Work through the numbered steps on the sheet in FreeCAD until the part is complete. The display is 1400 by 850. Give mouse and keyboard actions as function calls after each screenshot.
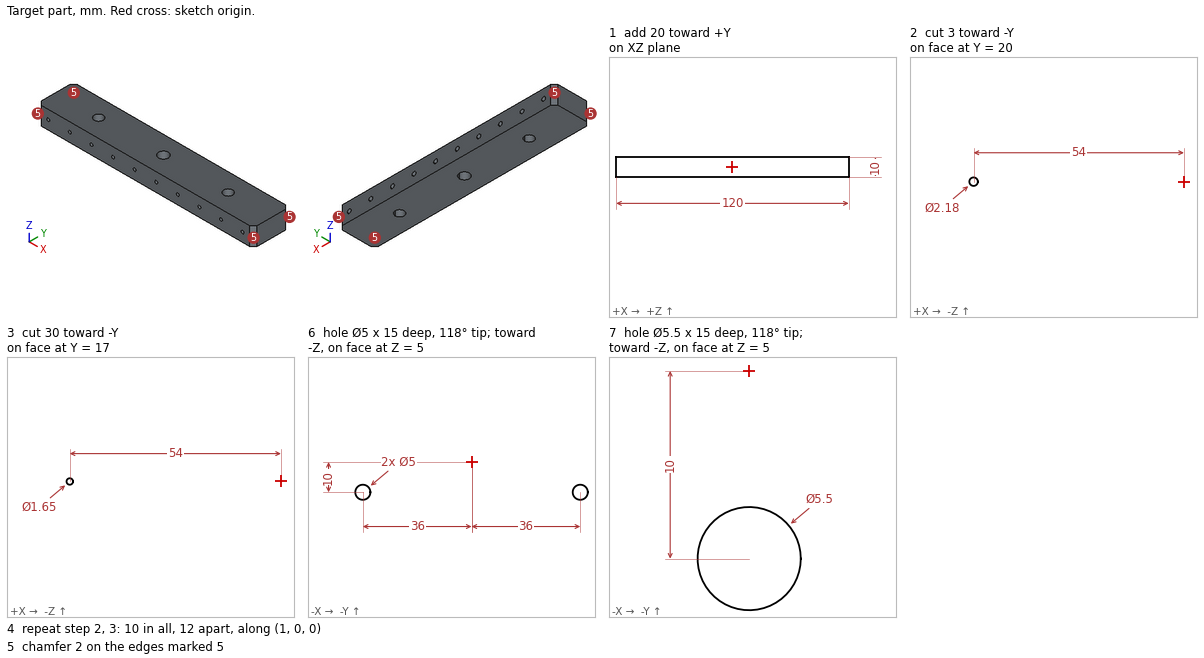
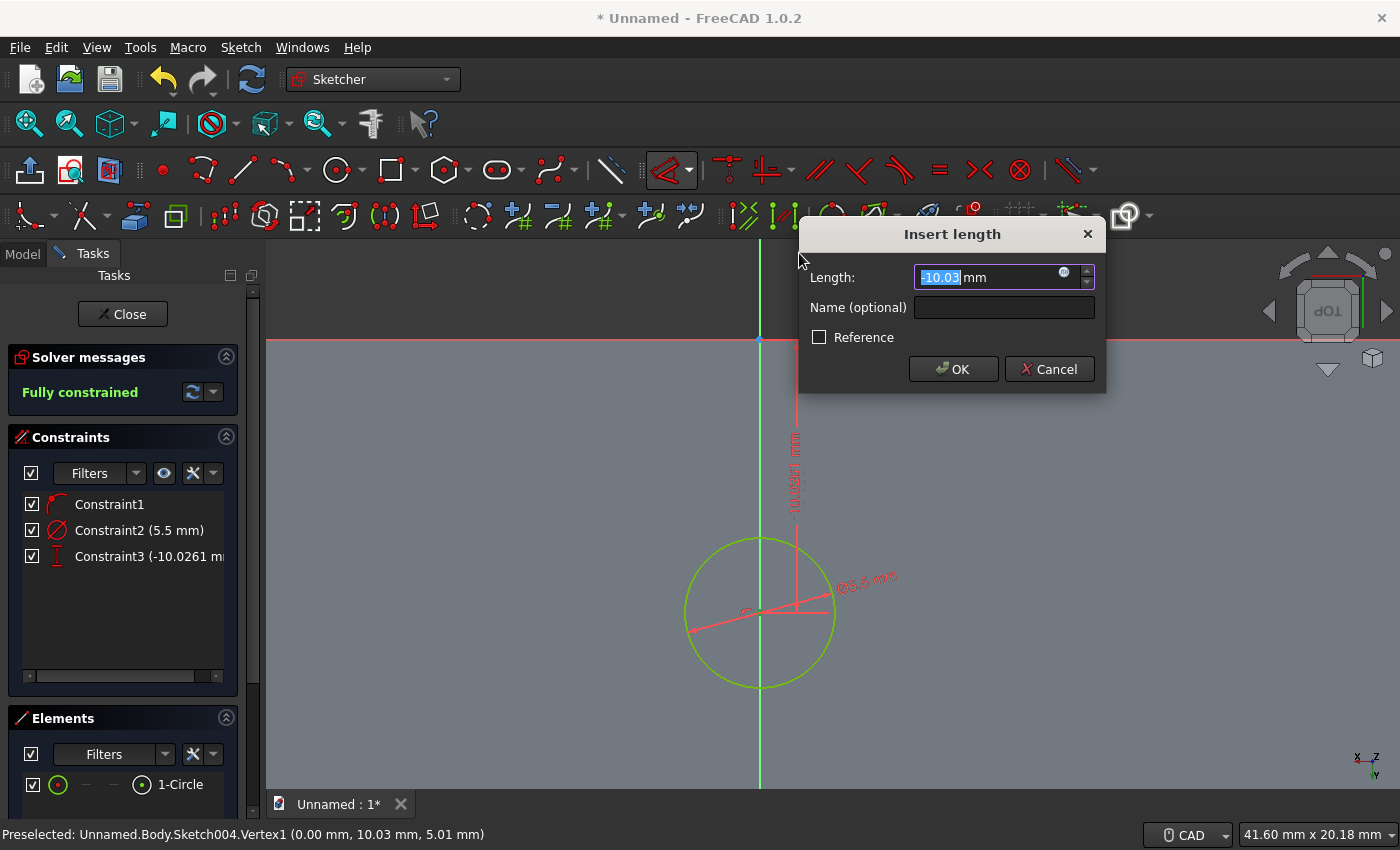
text(-10)
key(Return)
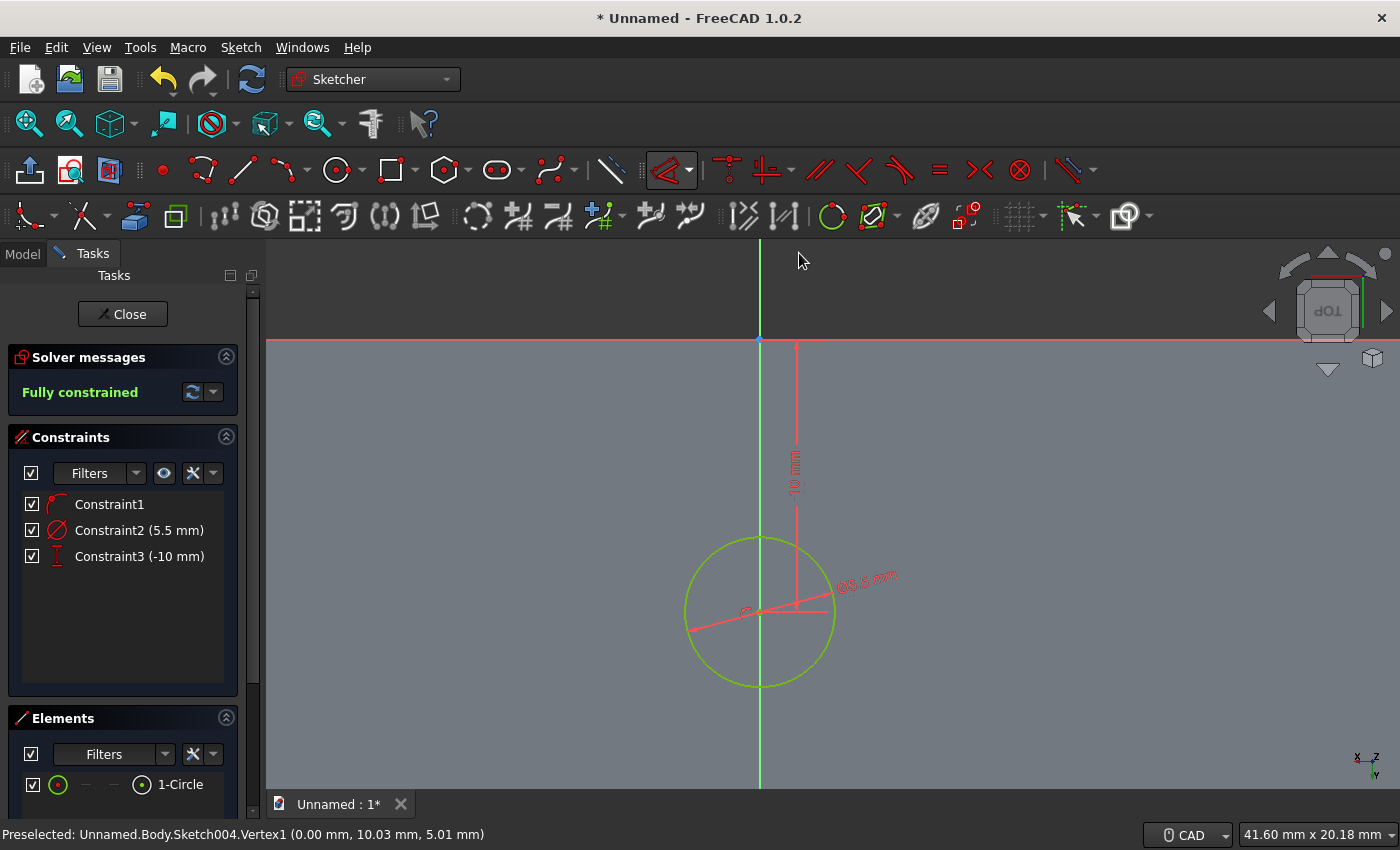
click(123, 314)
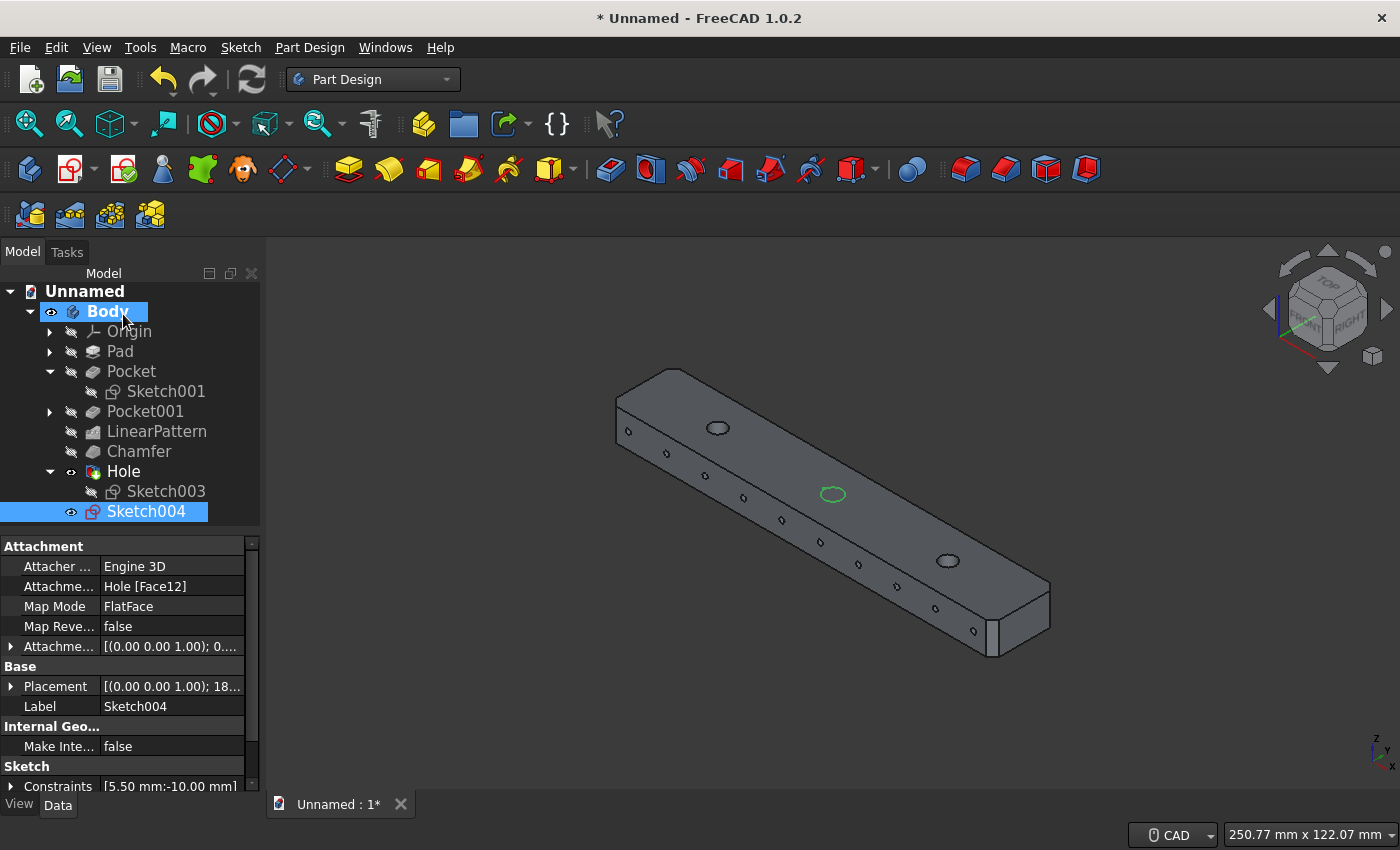
click(652, 170)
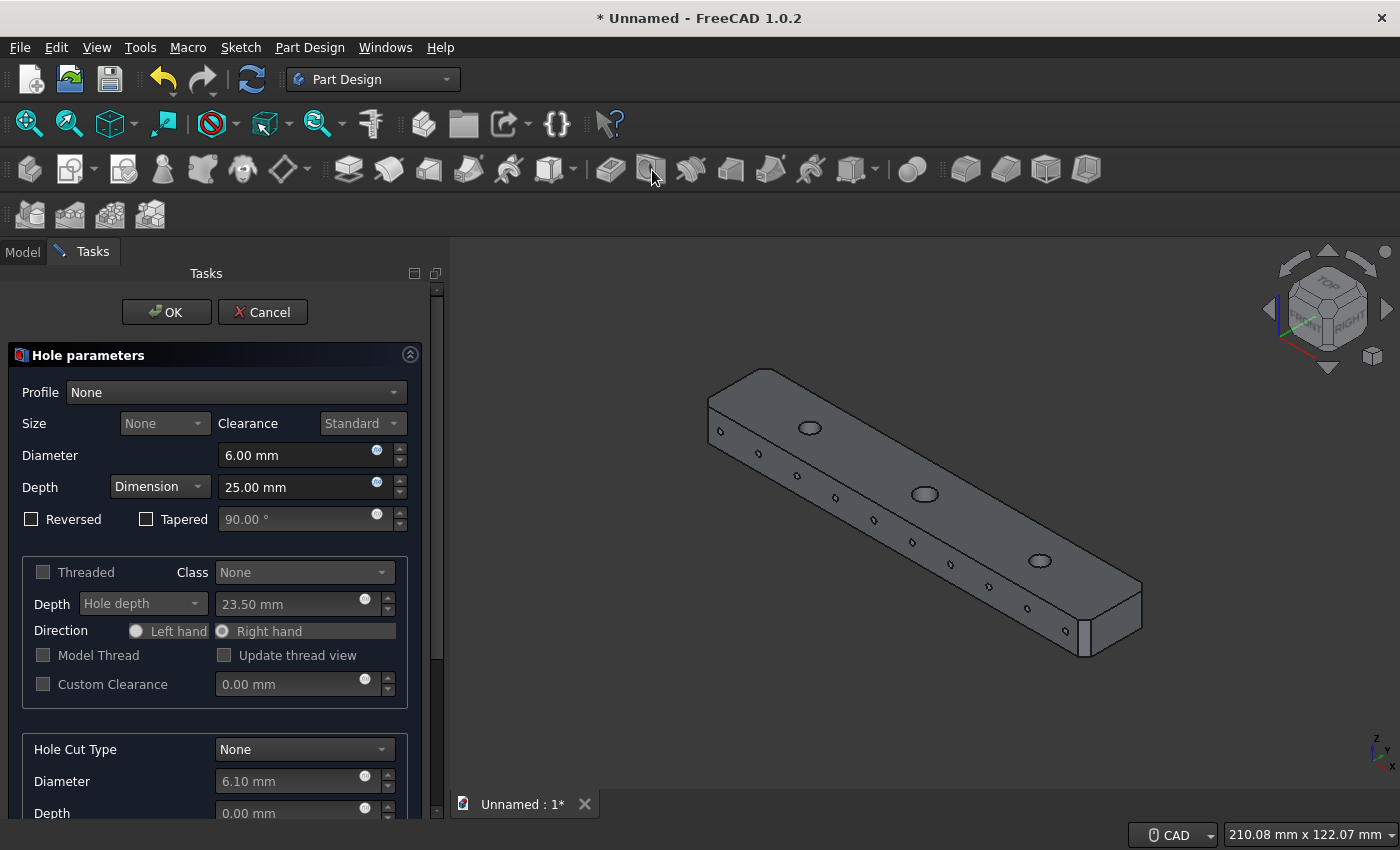
triple_click(305, 455)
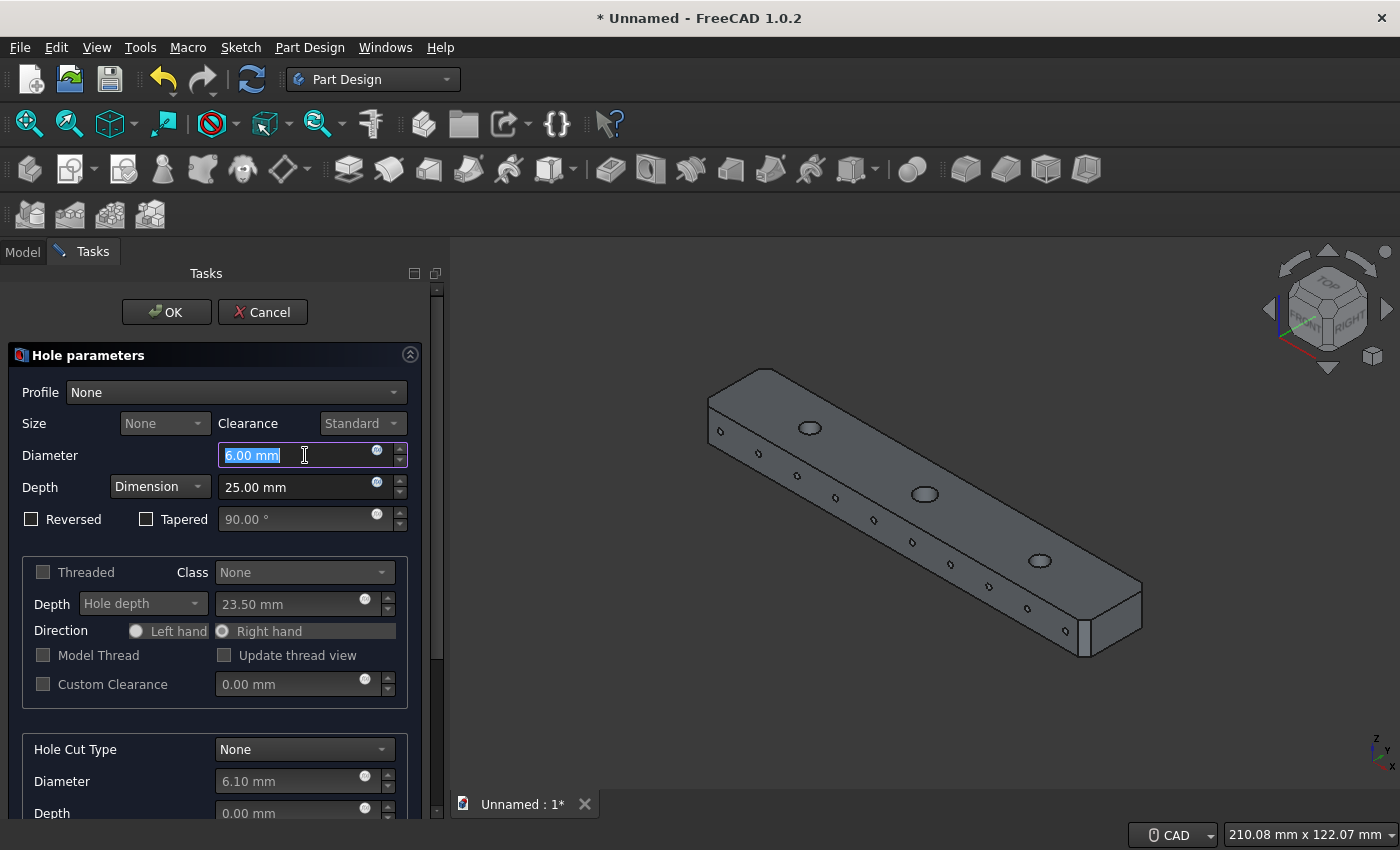
text(5.5)
key(Tab)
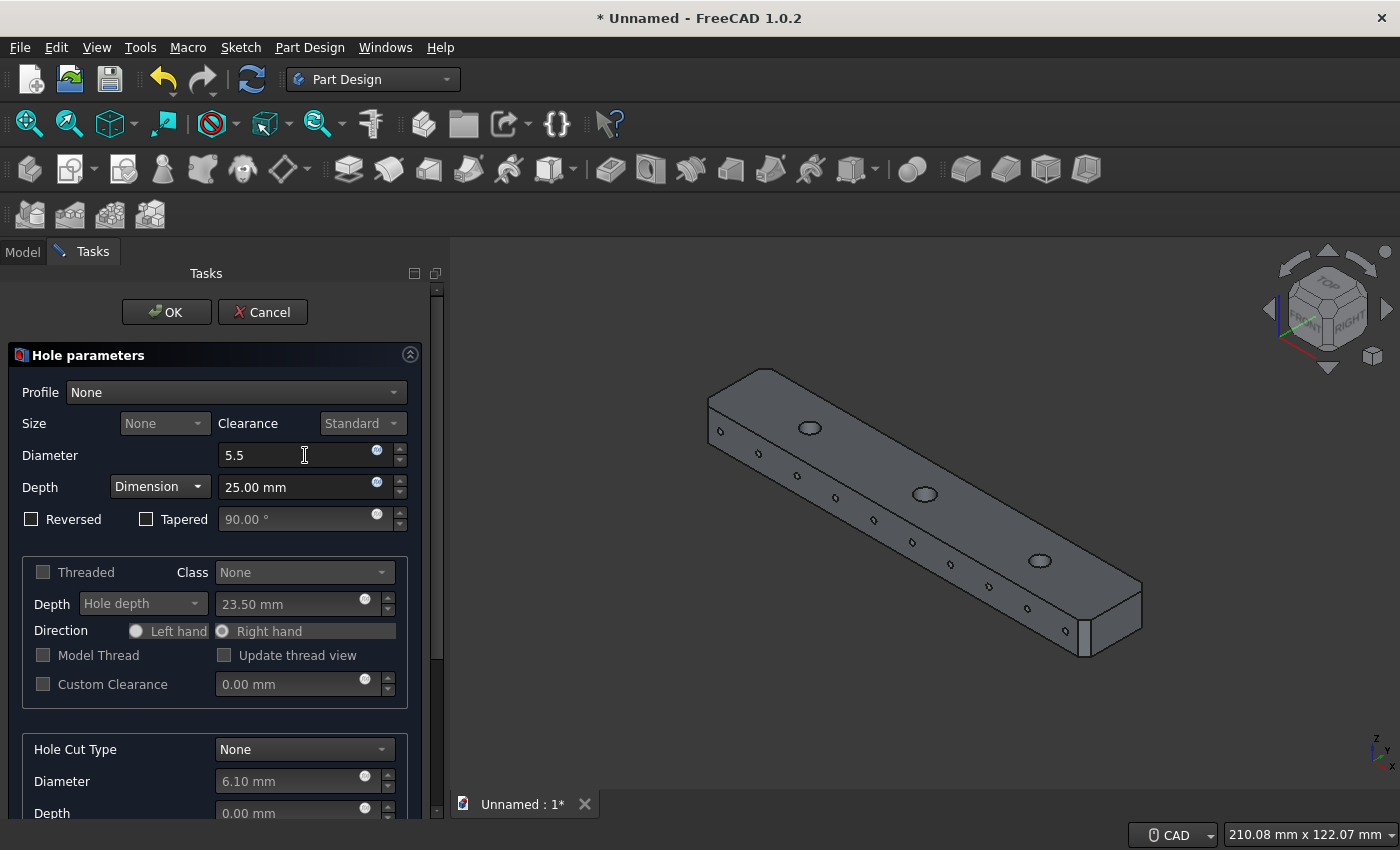
triple_click(305, 487)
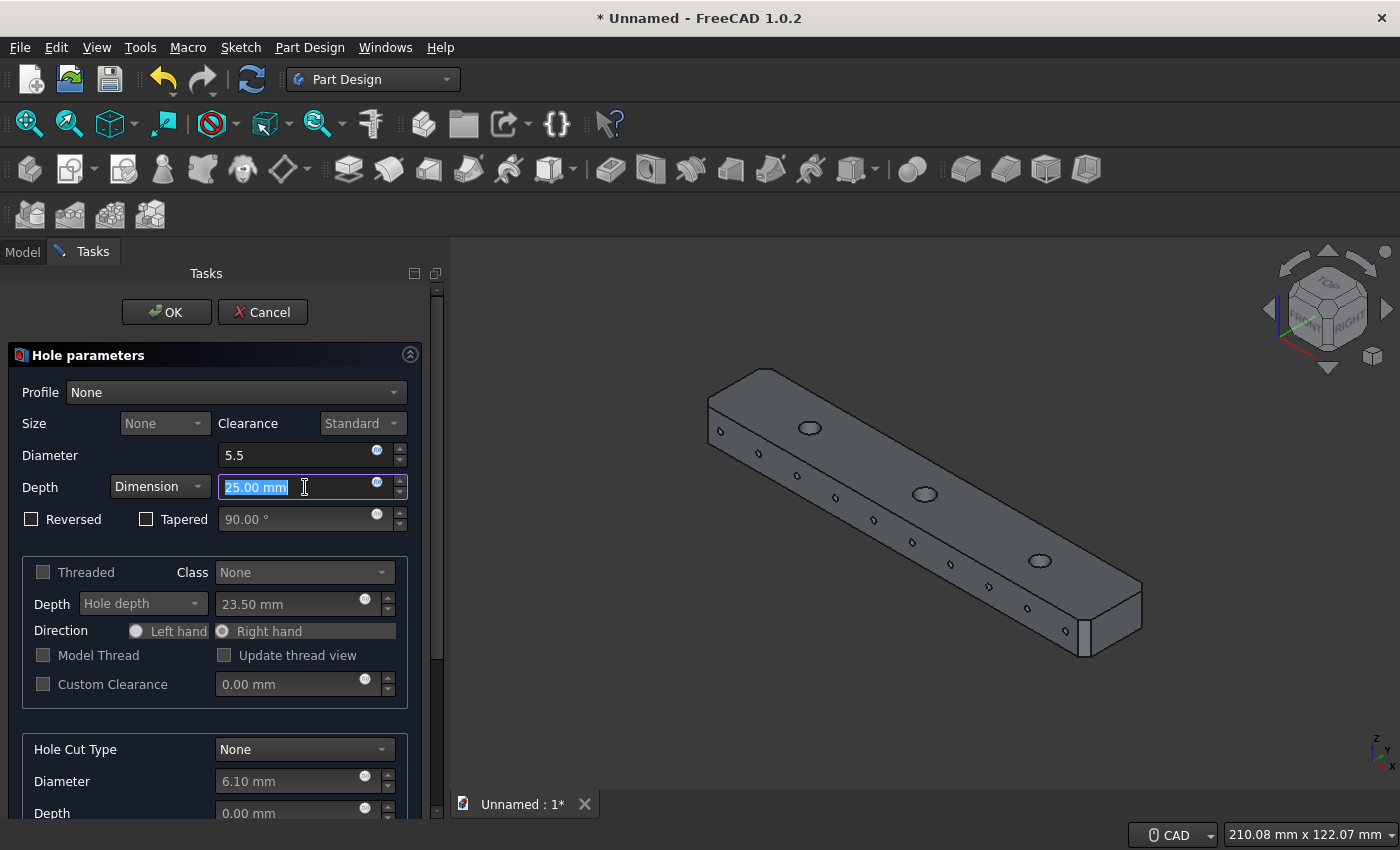
text(15)
key(Tab)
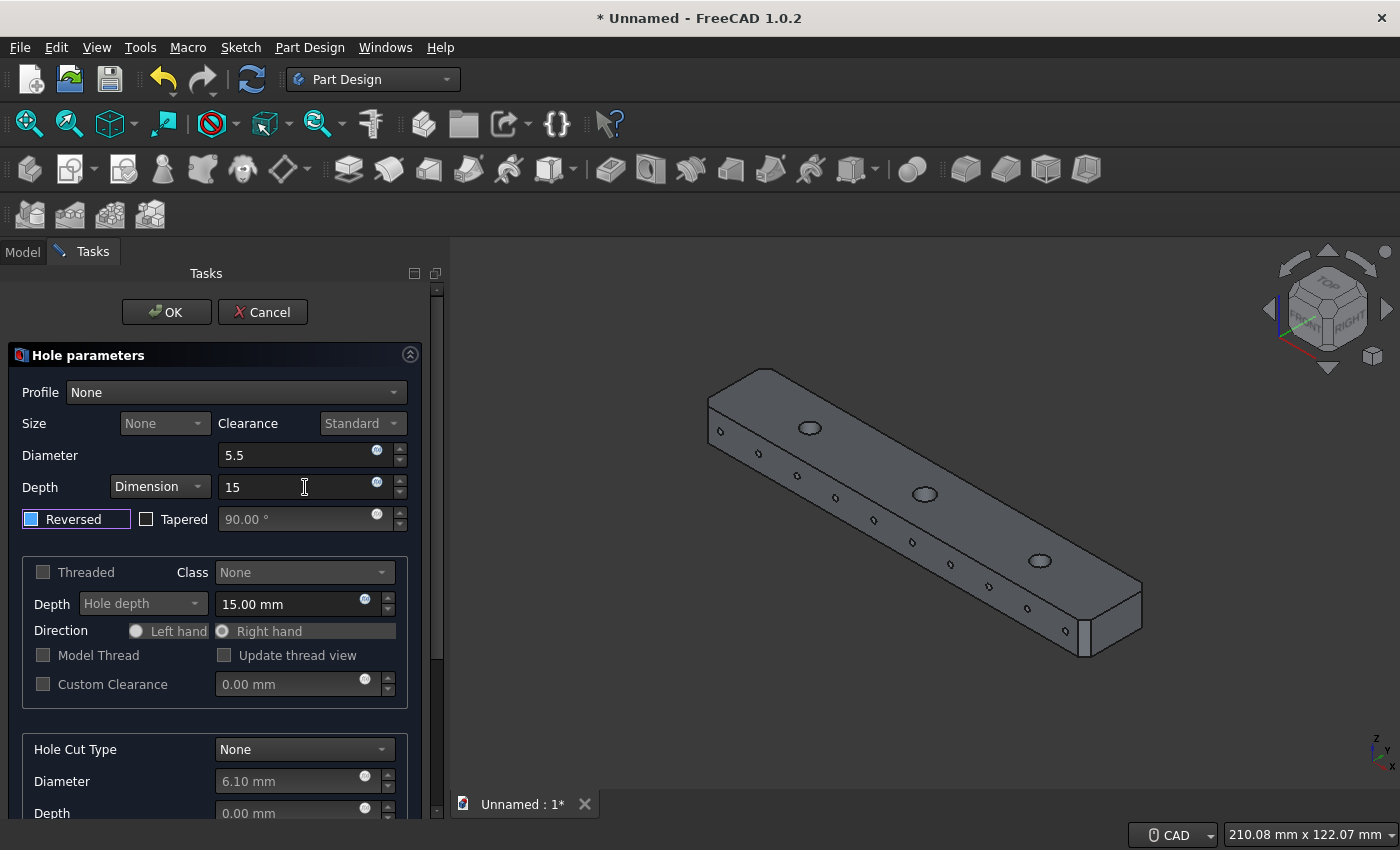
click(167, 312)